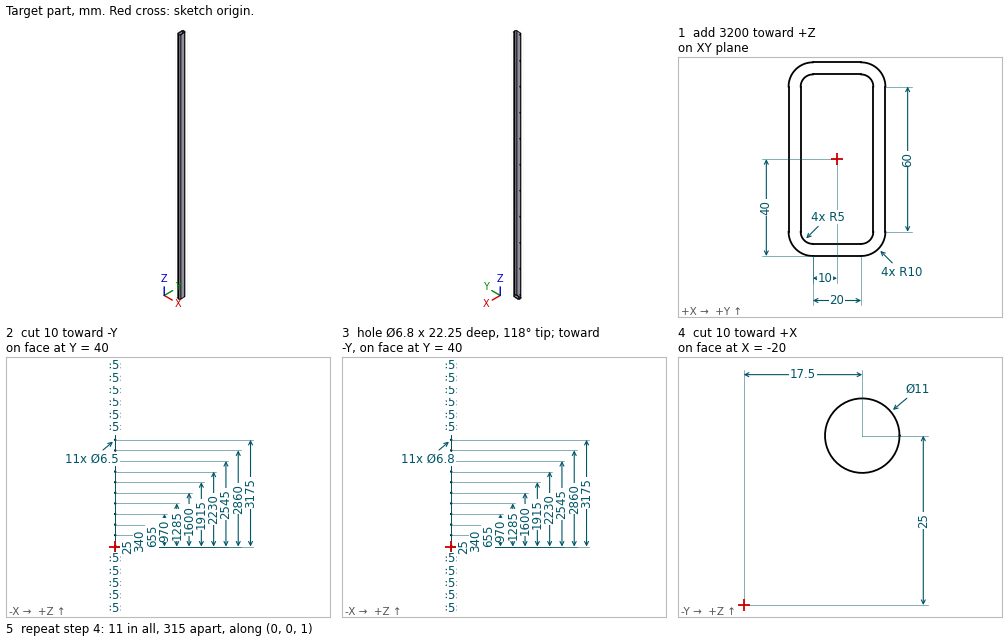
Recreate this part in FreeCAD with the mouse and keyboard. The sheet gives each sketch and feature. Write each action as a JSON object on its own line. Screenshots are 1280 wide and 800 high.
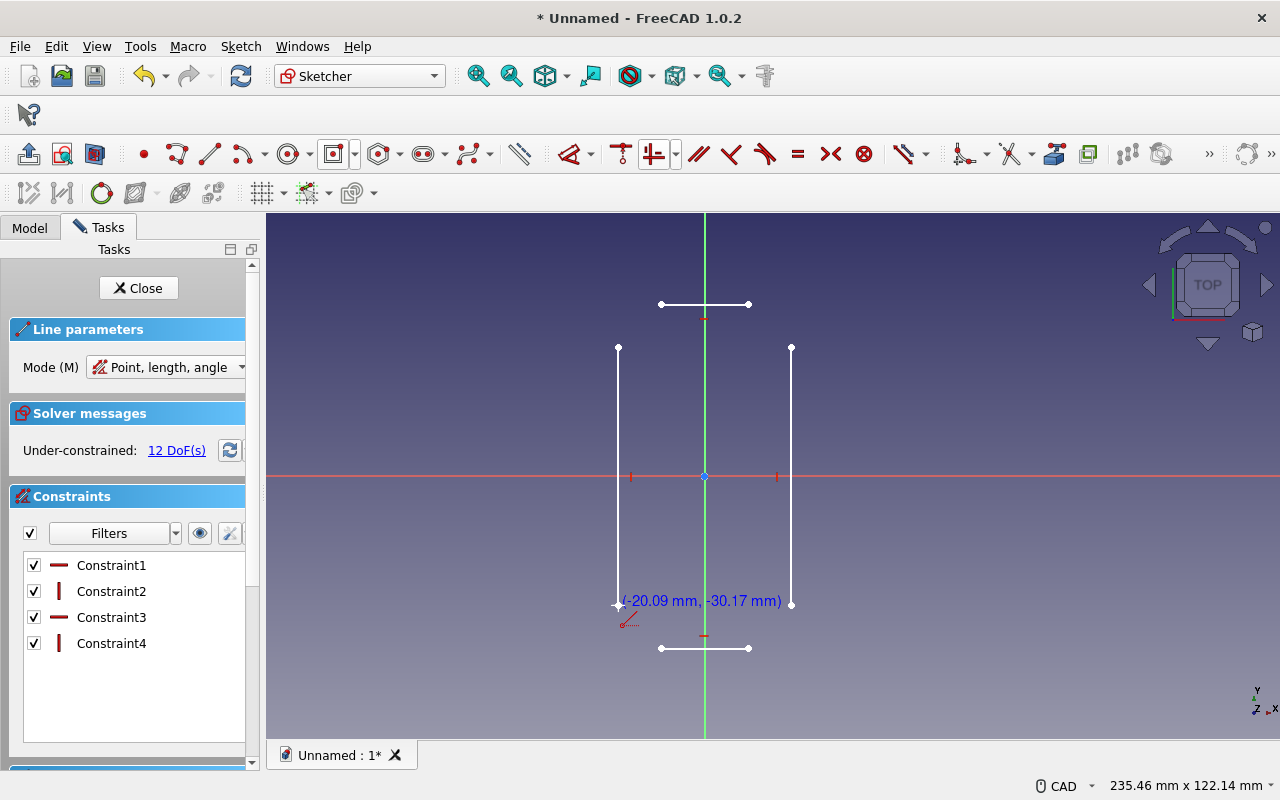
{"action": "key", "text": "g 3 a"}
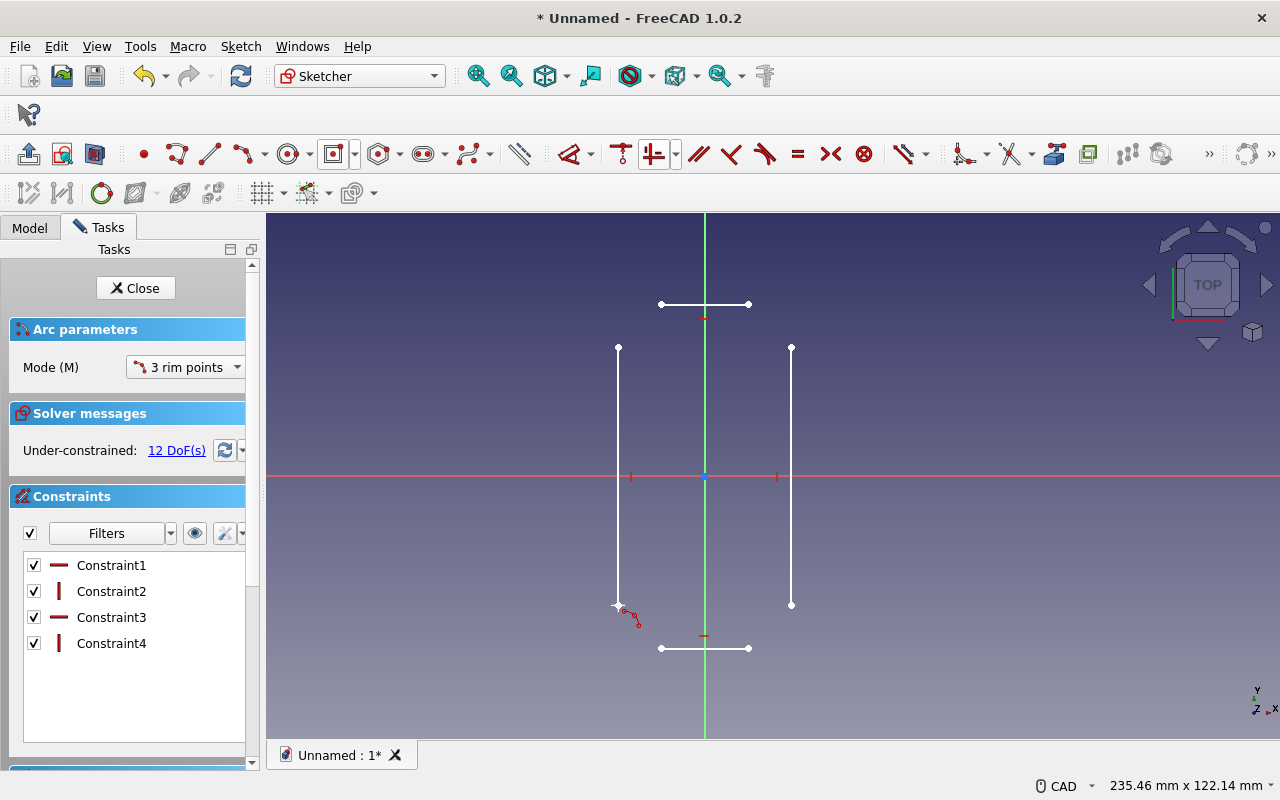
{"action": "left_click", "coordinate": [748, 649]}
{"action": "left_click", "coordinate": [791, 606]}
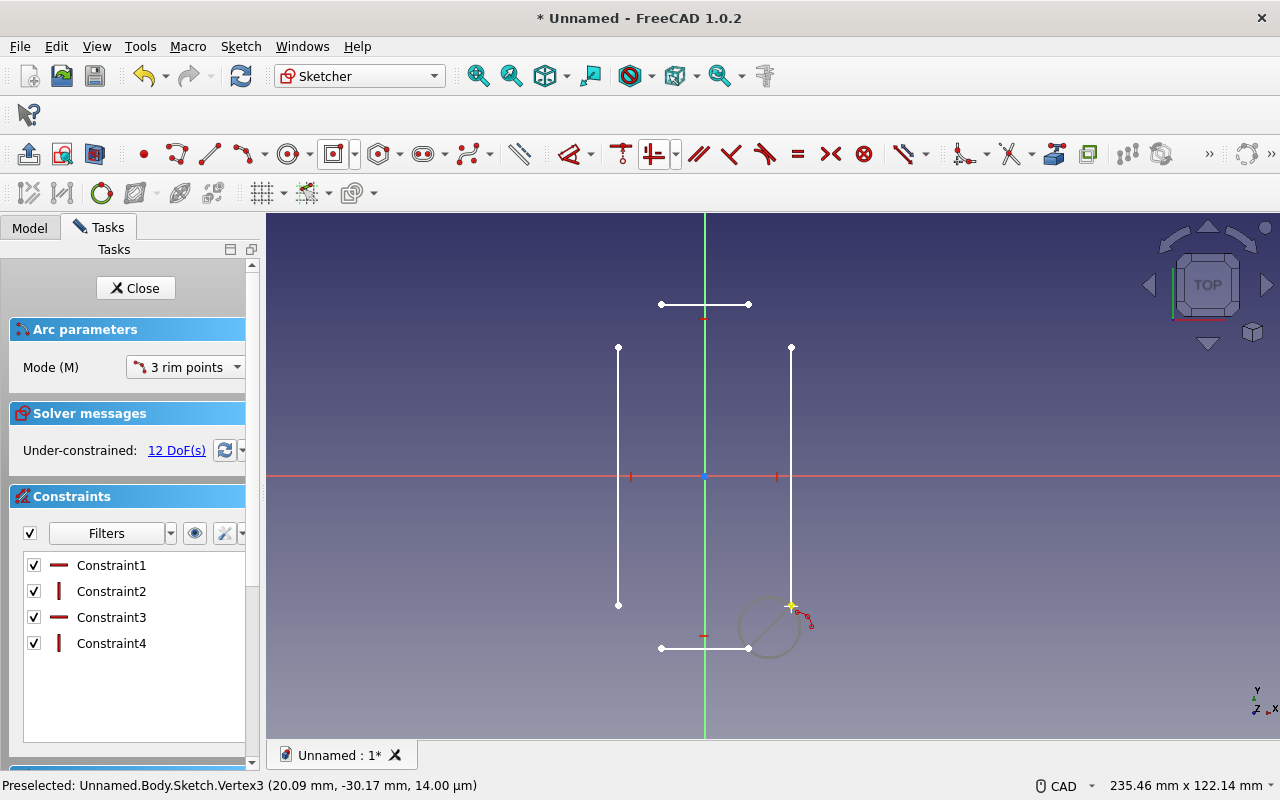
{"action": "scroll", "coordinate": [778, 636], "scroll_direction": "up", "scroll_amount": 2}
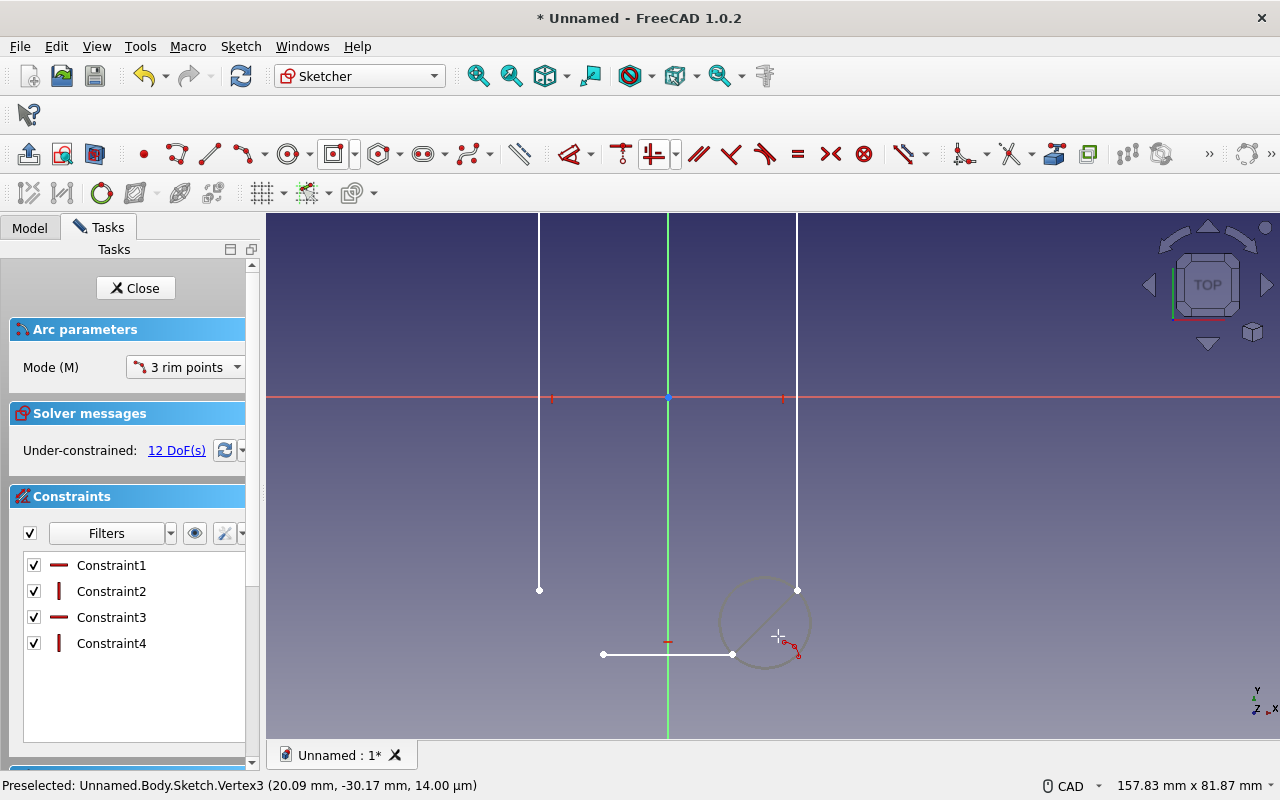
{"action": "left_click", "coordinate": [778, 635]}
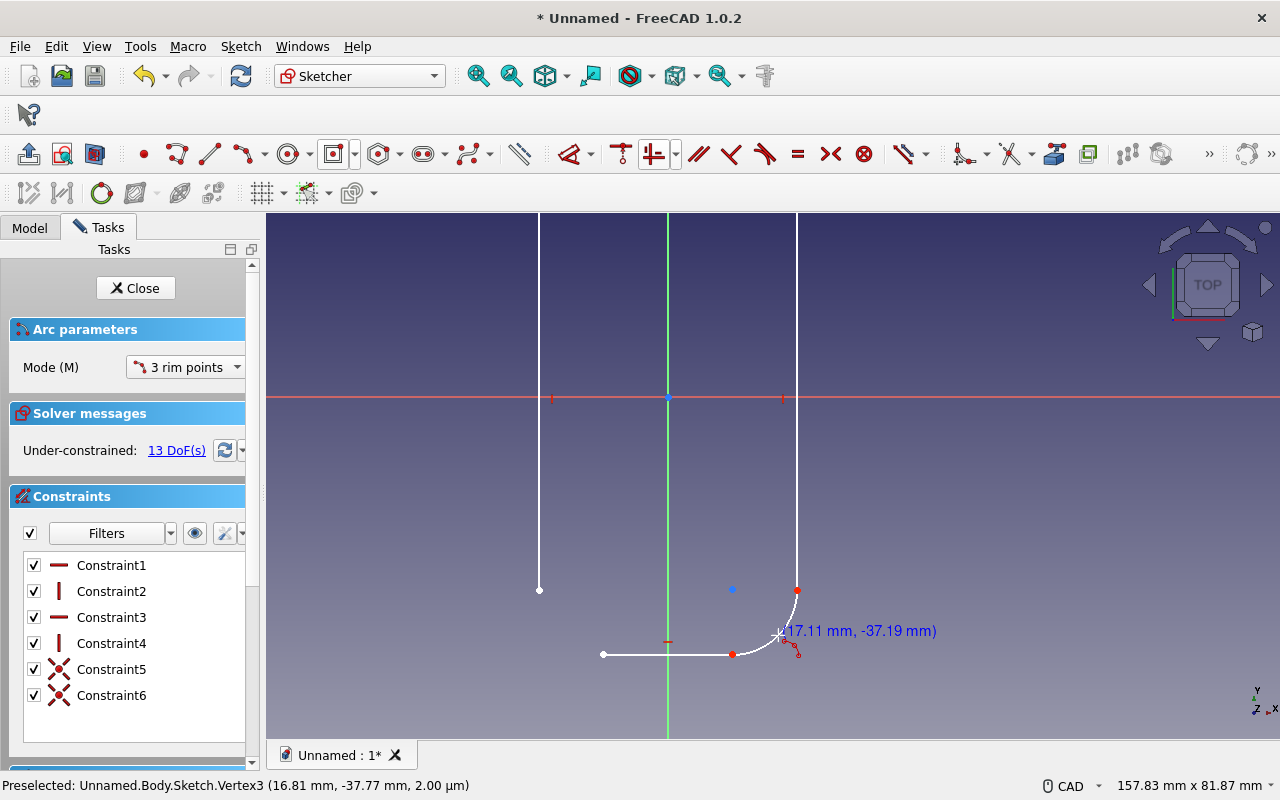
{"action": "scroll", "coordinate": [778, 637], "scroll_direction": "down", "scroll_amount": 2}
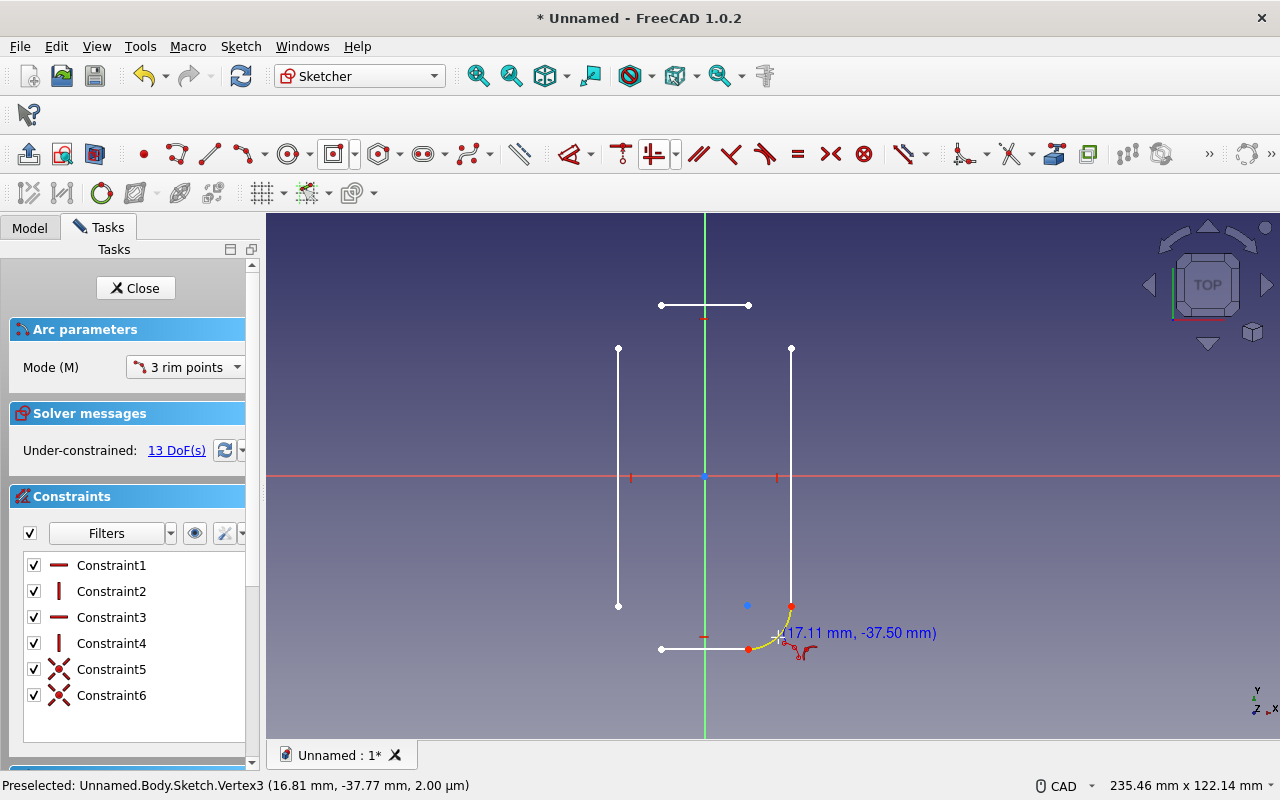
{"action": "left_click", "coordinate": [791, 348]}
{"action": "left_click", "coordinate": [748, 305]}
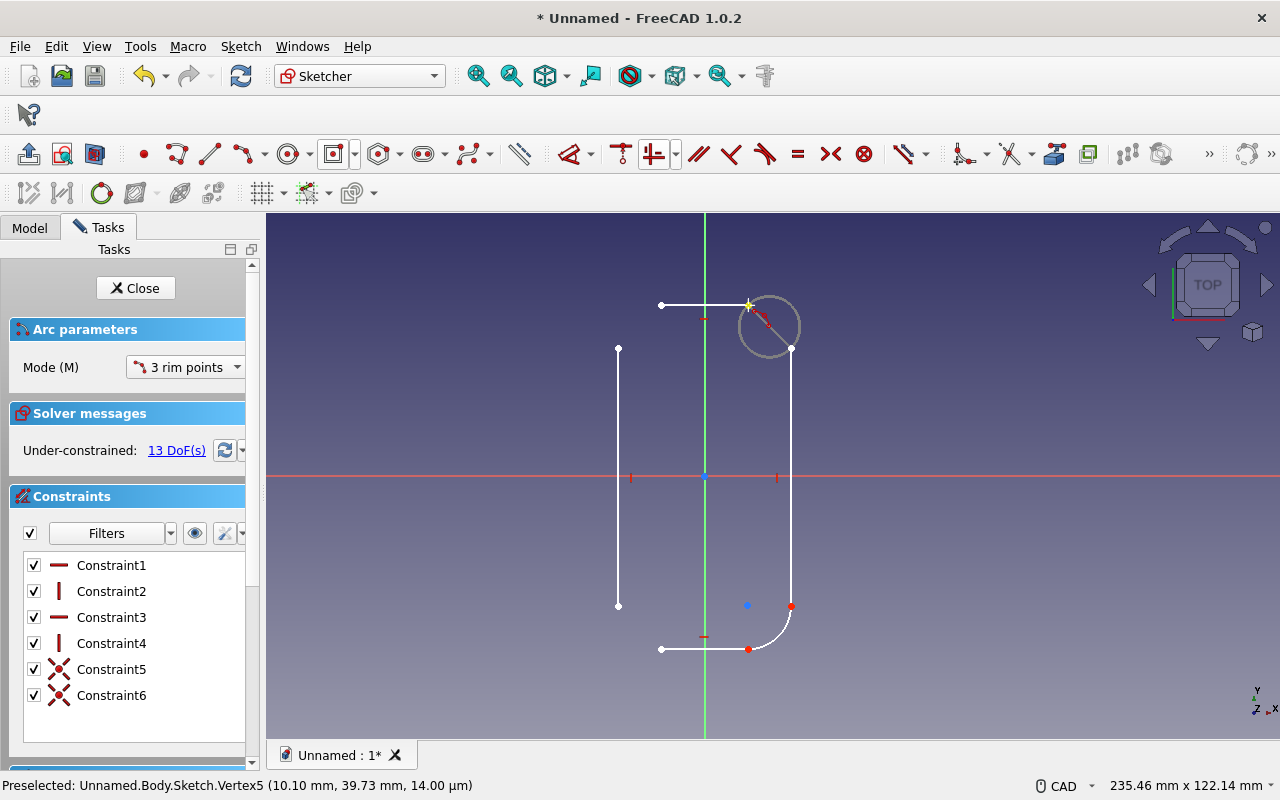
{"action": "scroll", "coordinate": [778, 317], "scroll_direction": "up", "scroll_amount": 2}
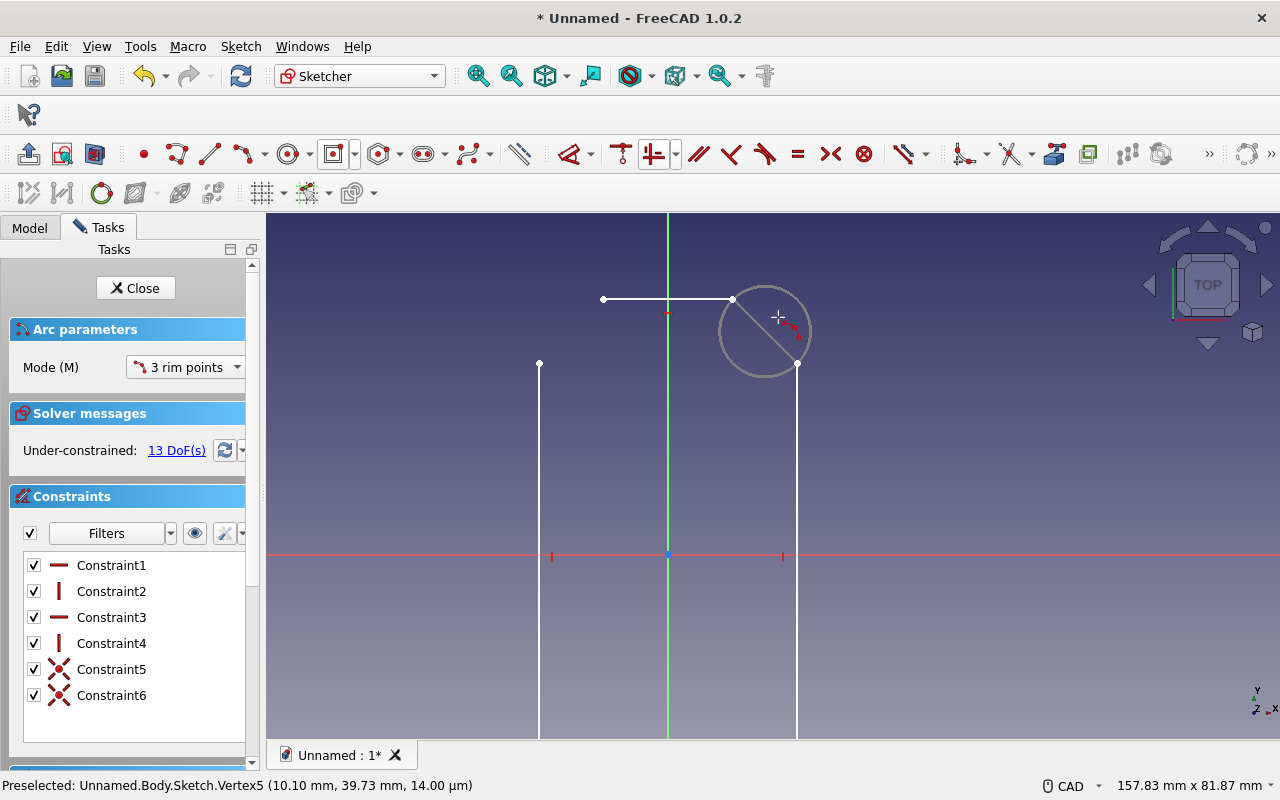
{"action": "left_click", "coordinate": [778, 317]}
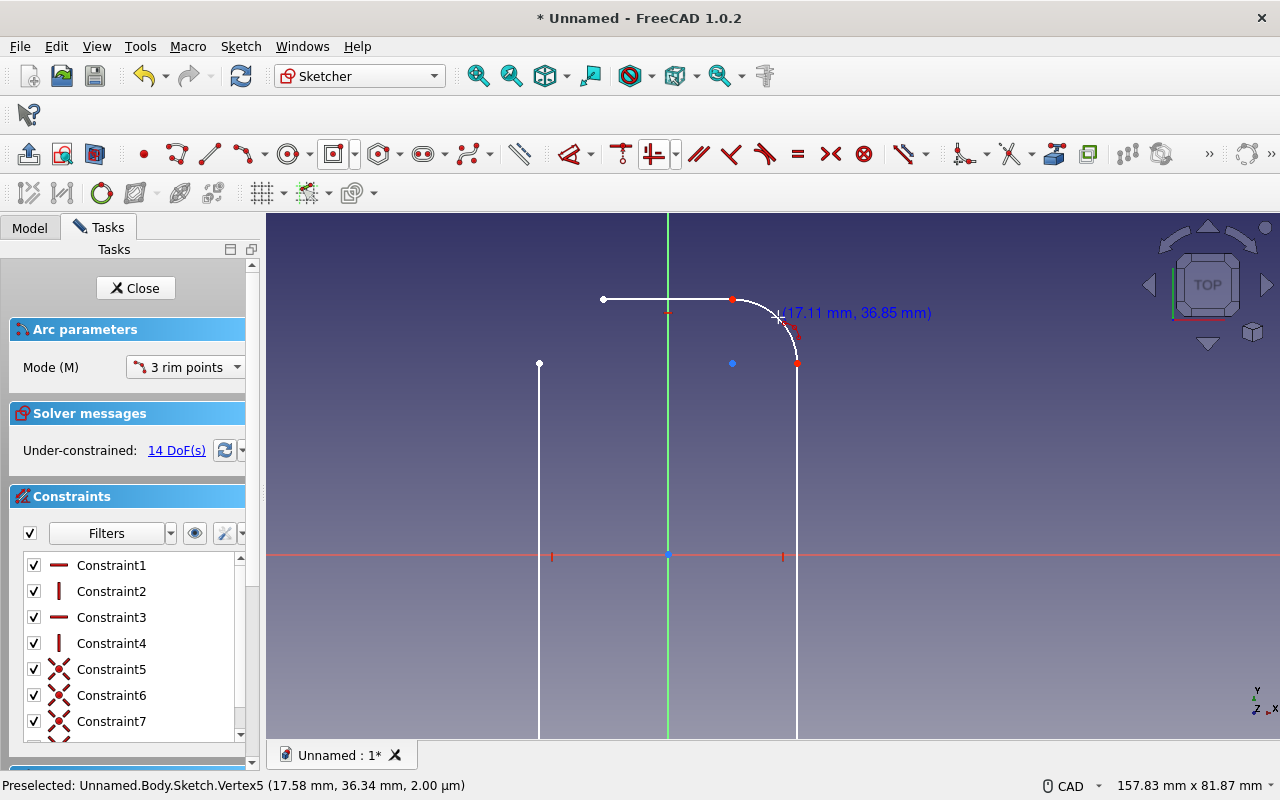
{"action": "left_click", "coordinate": [603, 299]}
{"action": "left_click", "coordinate": [539, 364]}
{"action": "left_click", "coordinate": [558, 317]}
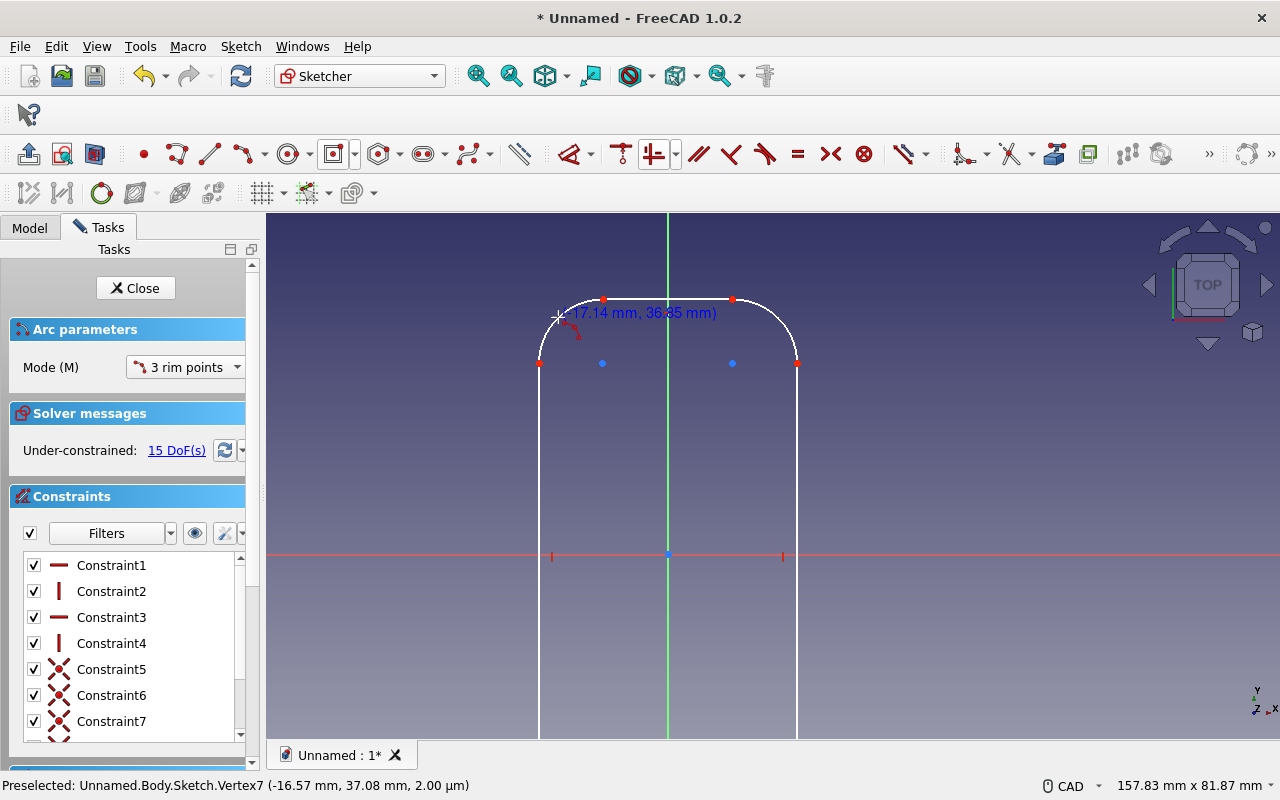
{"action": "scroll", "coordinate": [778, 316], "scroll_direction": "down", "scroll_amount": 2}